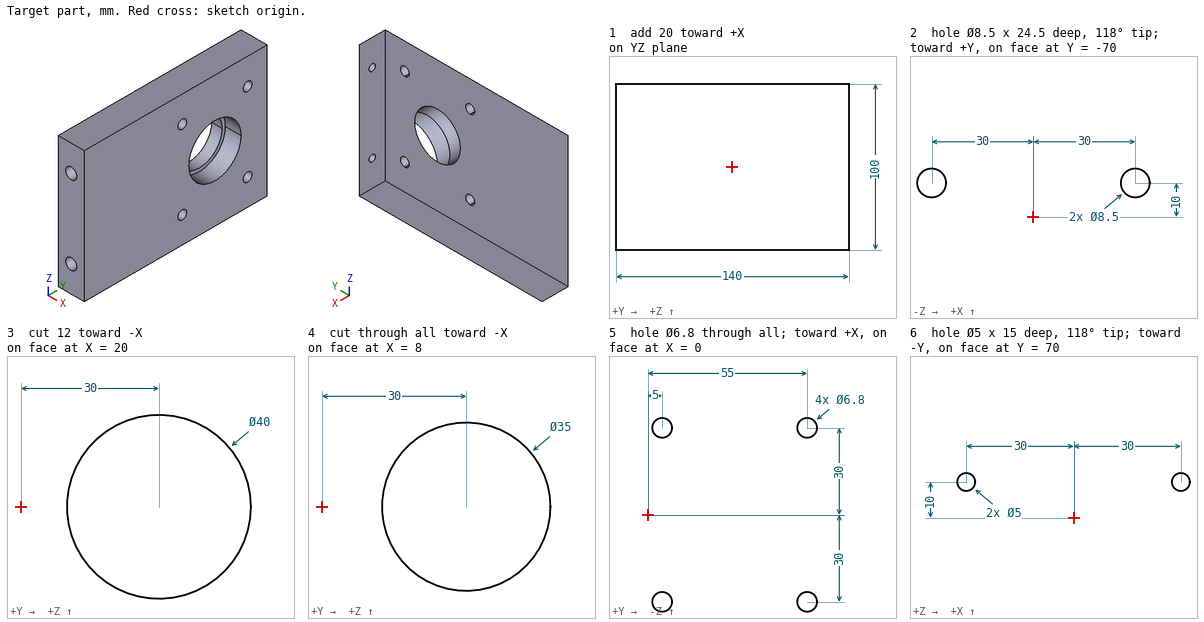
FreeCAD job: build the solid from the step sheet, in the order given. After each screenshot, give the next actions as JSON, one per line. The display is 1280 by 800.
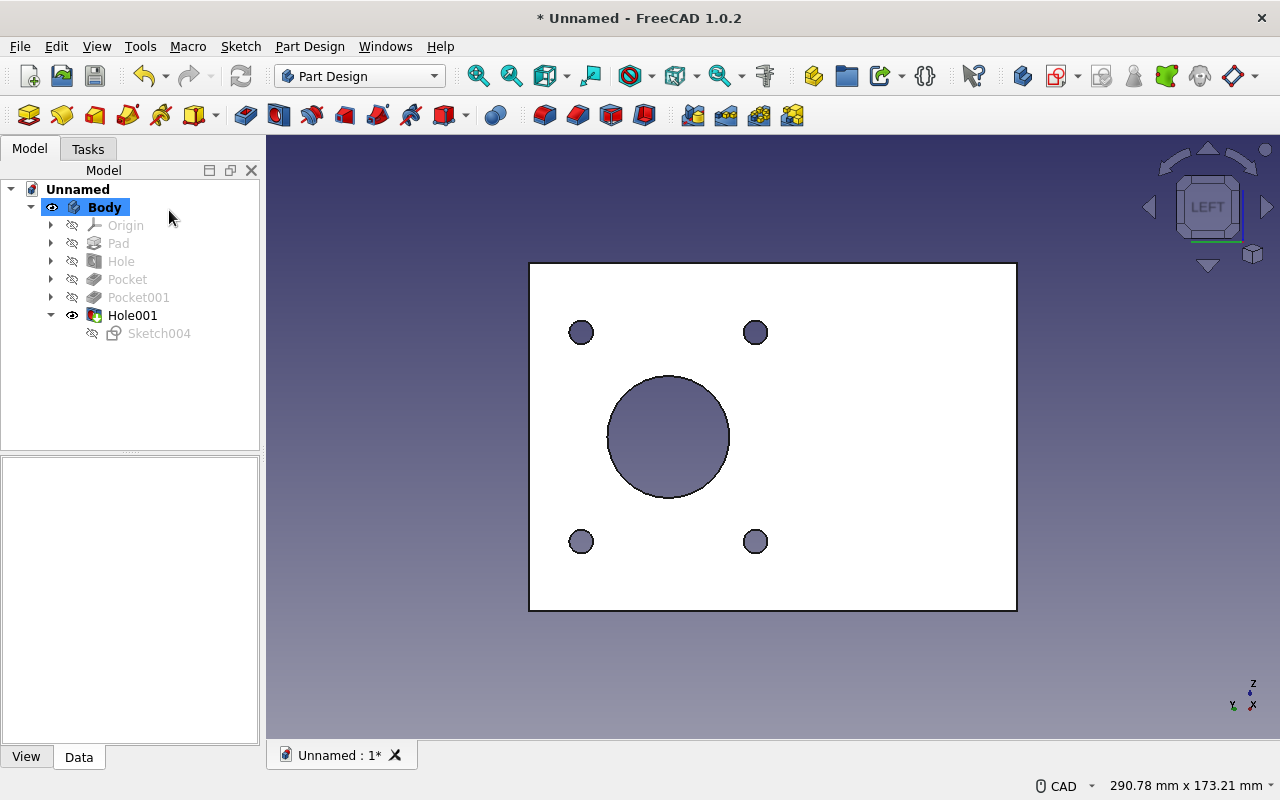
{"action": "key", "text": "4"}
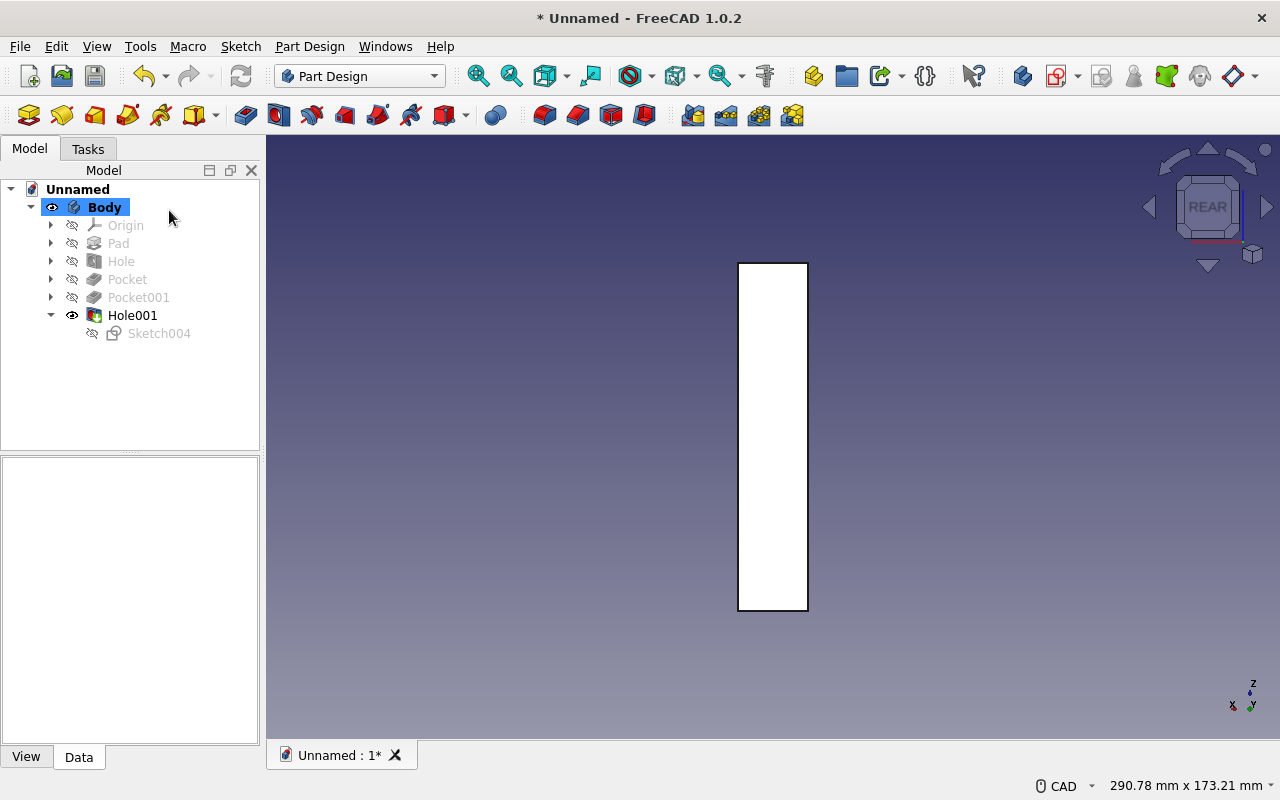
{"action": "left_click", "coordinate": [773, 436]}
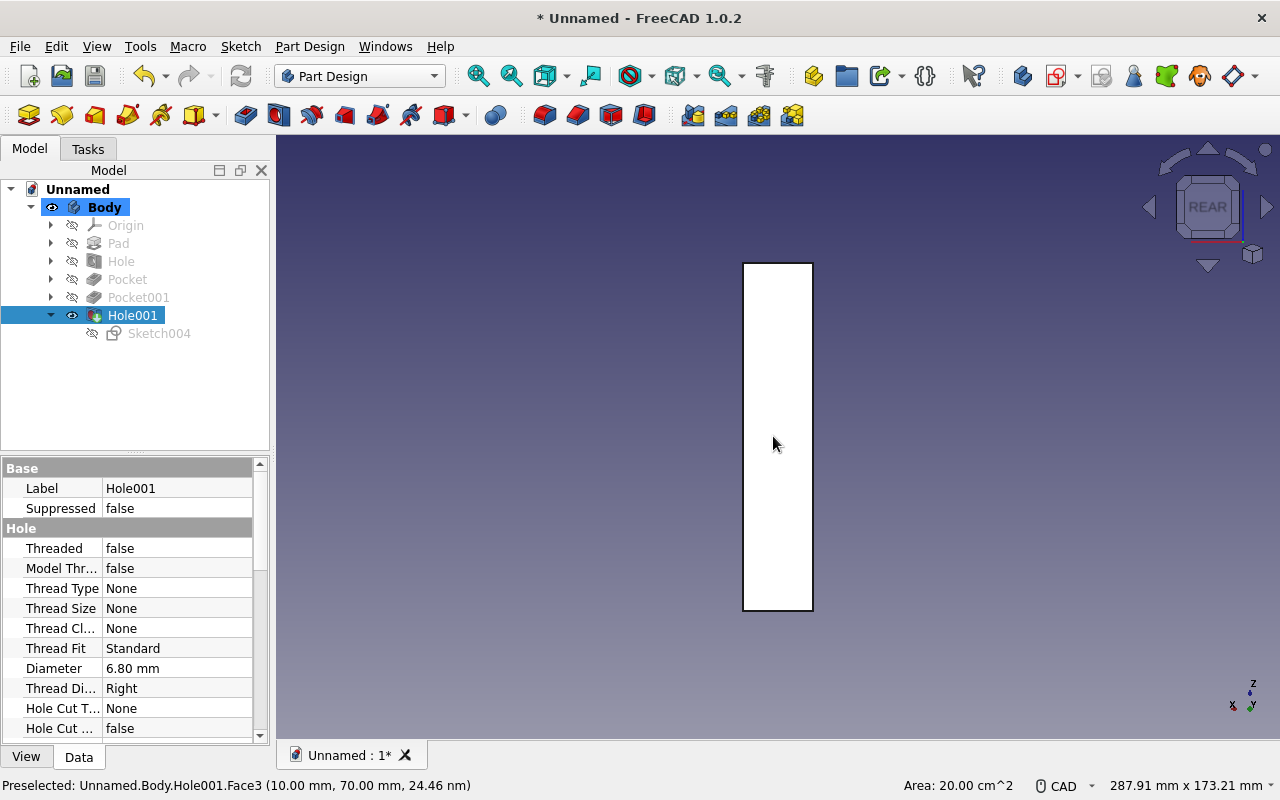
{"action": "left_click", "coordinate": [1056, 76]}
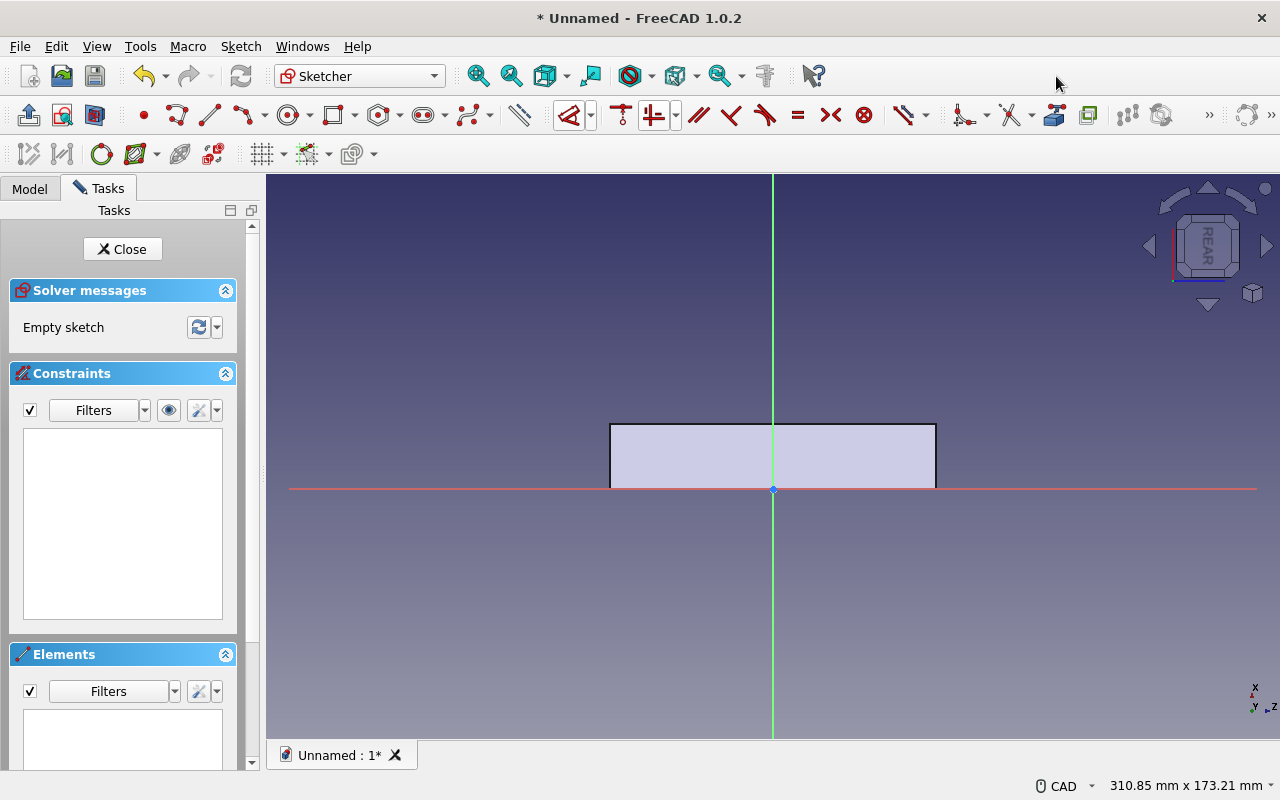
{"action": "scroll", "coordinate": [813, 476], "scroll_direction": "up", "scroll_amount": 5}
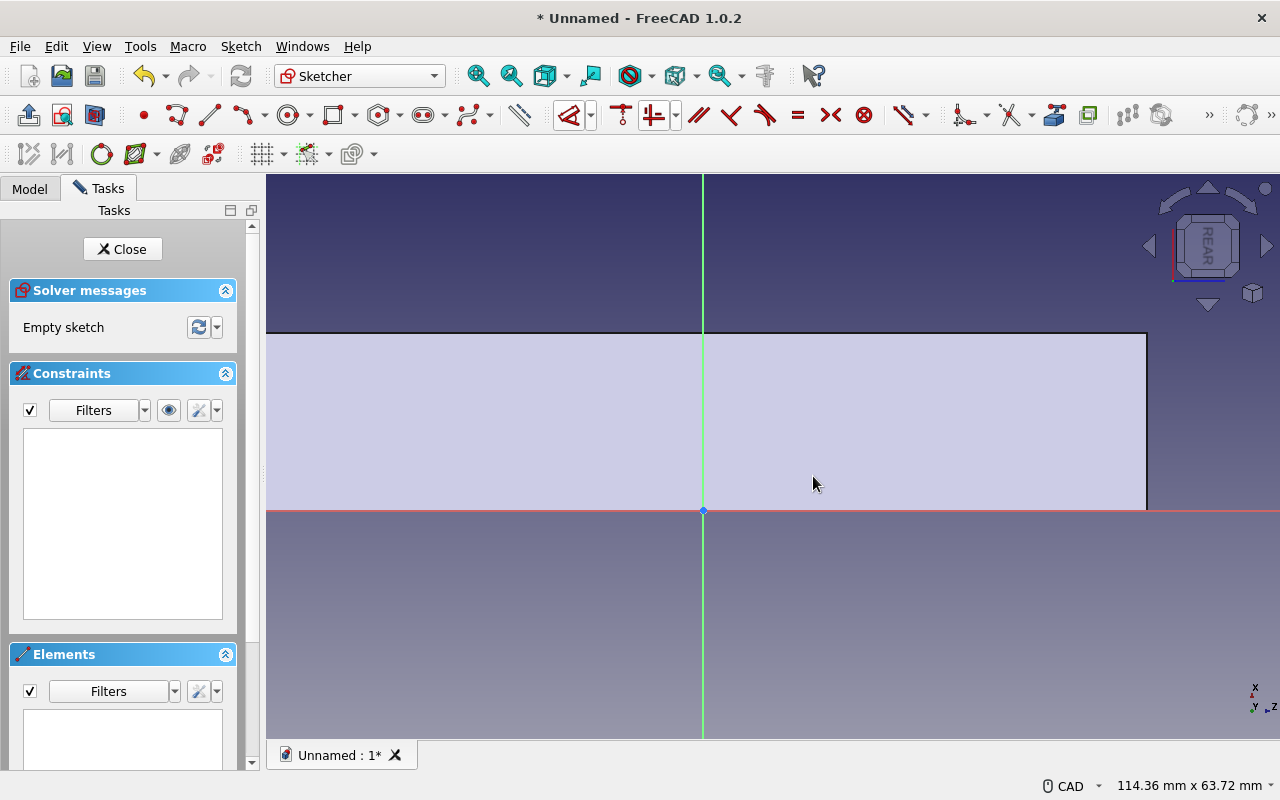
{"action": "left_click", "coordinate": [288, 116]}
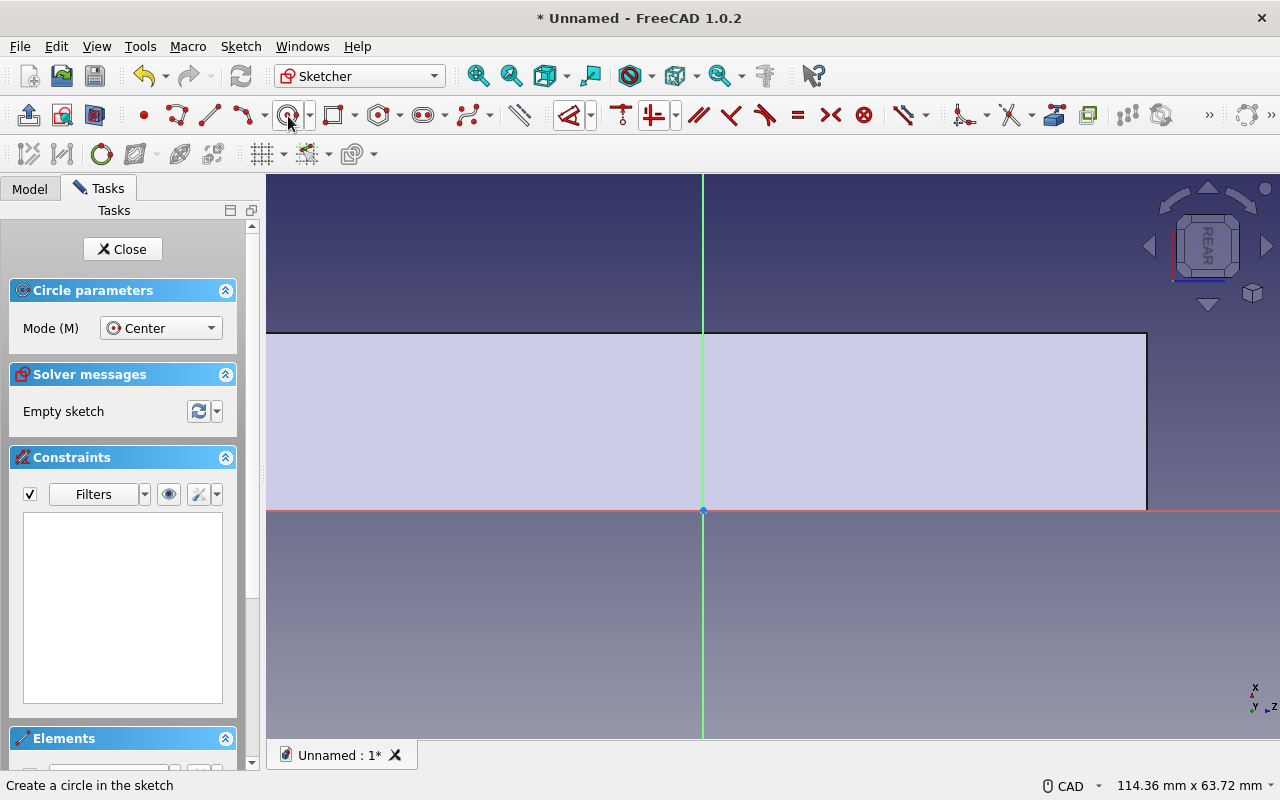
{"action": "left_click", "coordinate": [437, 422]}
{"action": "mouse_move", "coordinate": [453, 406]}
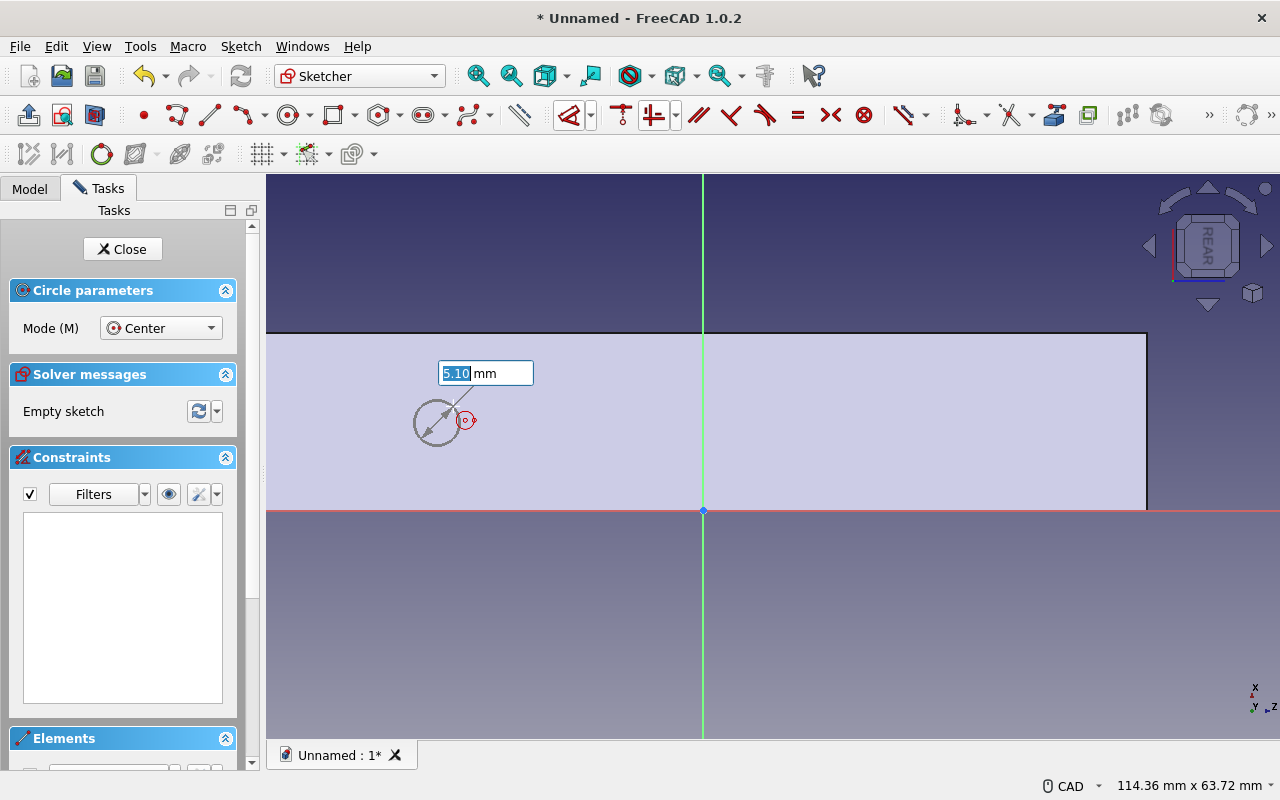
{"action": "type", "text": "5"}
{"action": "key", "text": "Return"}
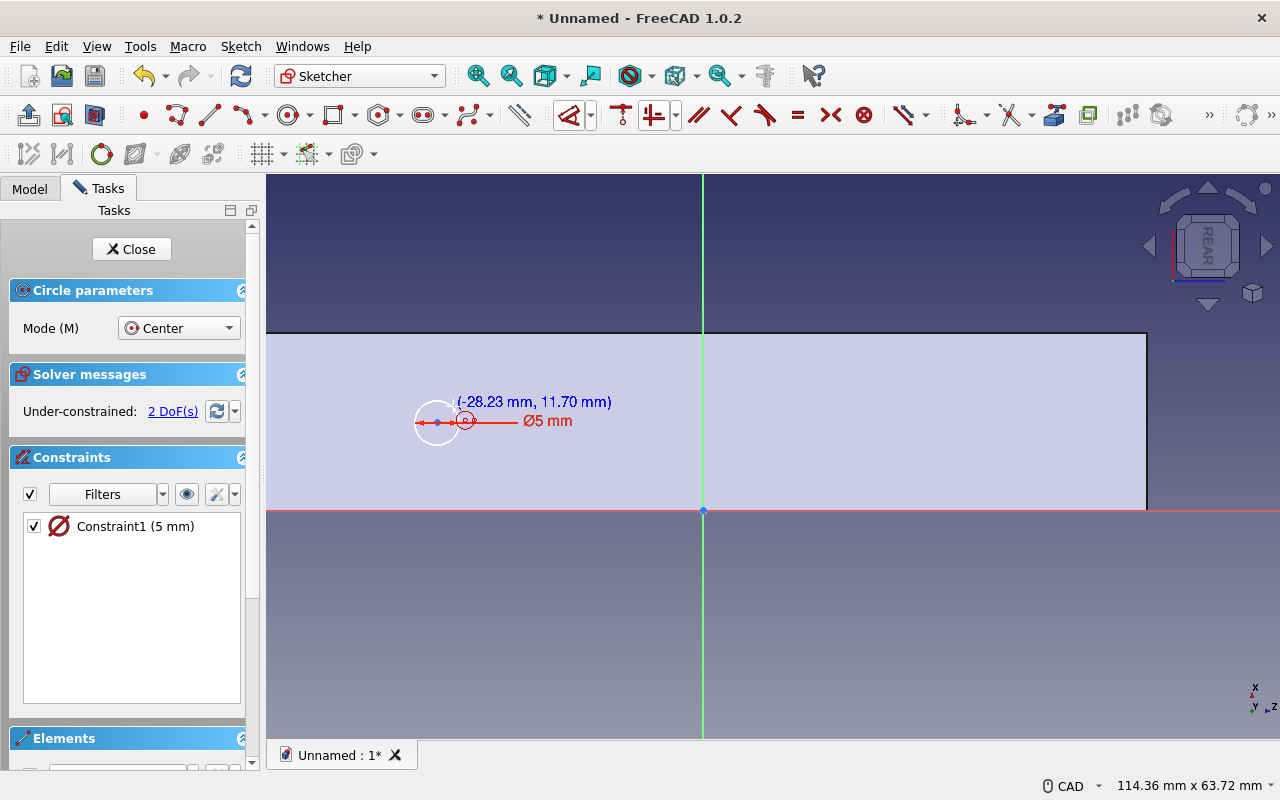
{"action": "left_click", "coordinate": [969, 422]}
{"action": "mouse_move", "coordinate": [985, 406]}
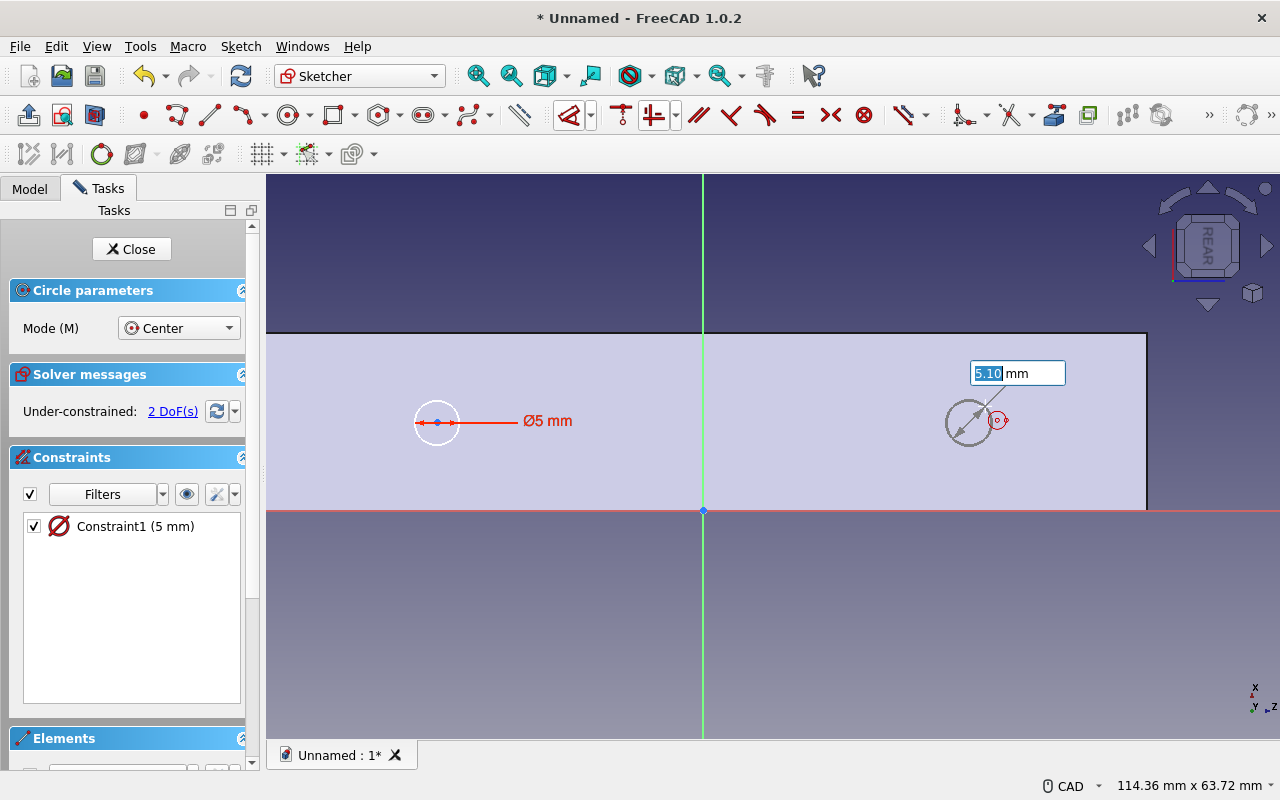
{"action": "type", "text": "5"}
{"action": "key", "text": "Return"}
{"action": "key", "text": "Escape"}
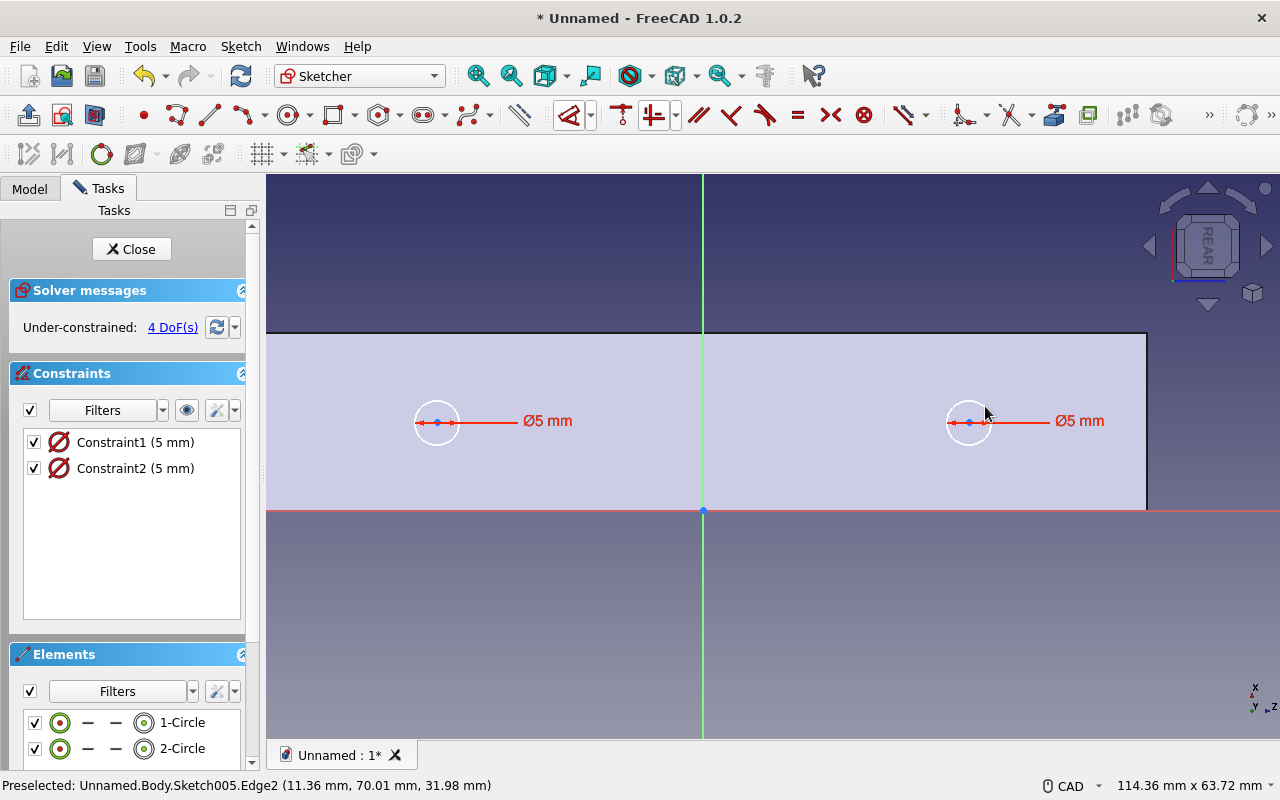
{"action": "left_click", "coordinate": [437, 423]}